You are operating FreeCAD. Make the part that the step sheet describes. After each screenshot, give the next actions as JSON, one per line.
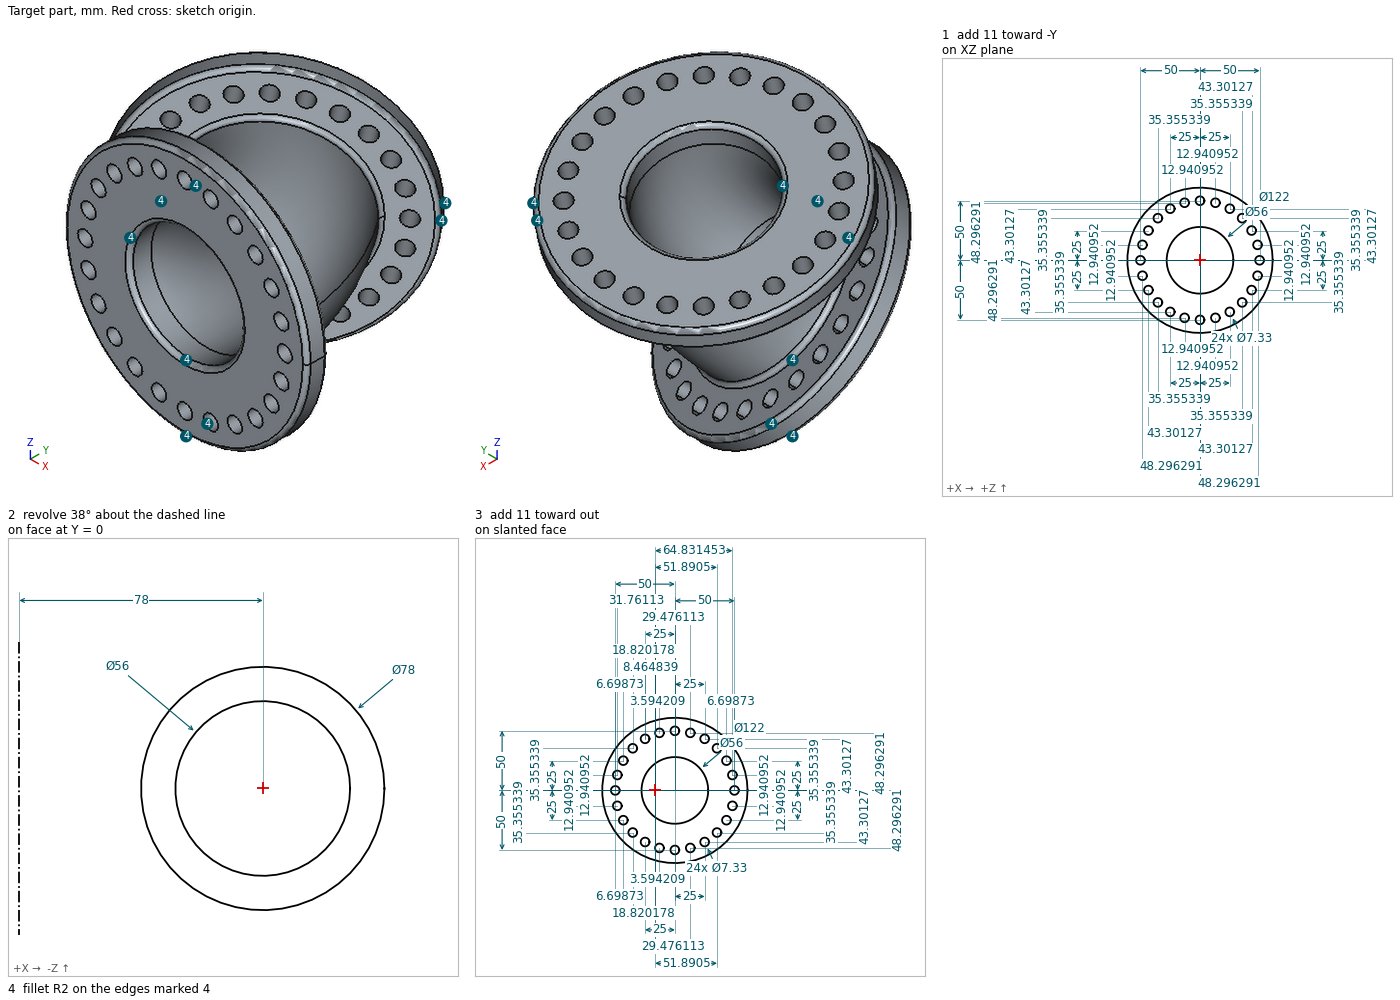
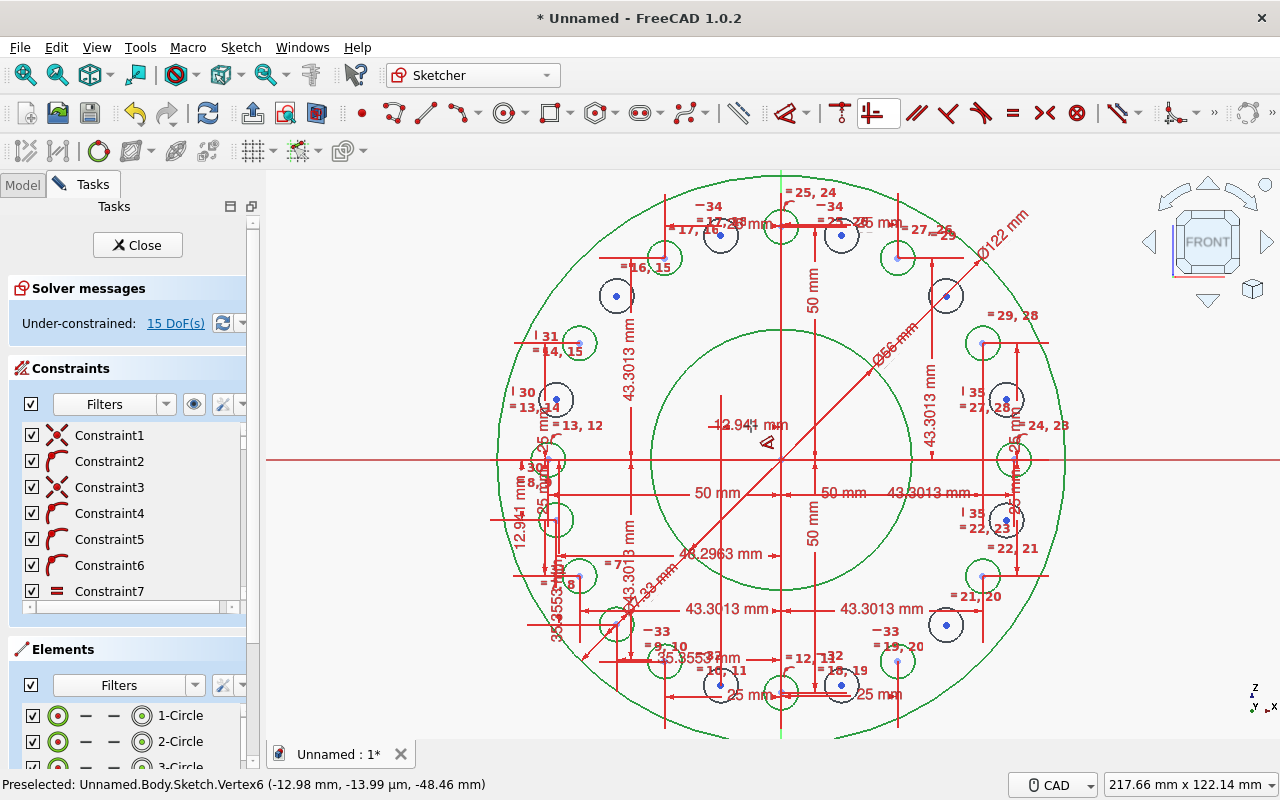
{"action": "left_click", "coordinate": [721, 686]}
{"action": "left_click", "coordinate": [687, 521]}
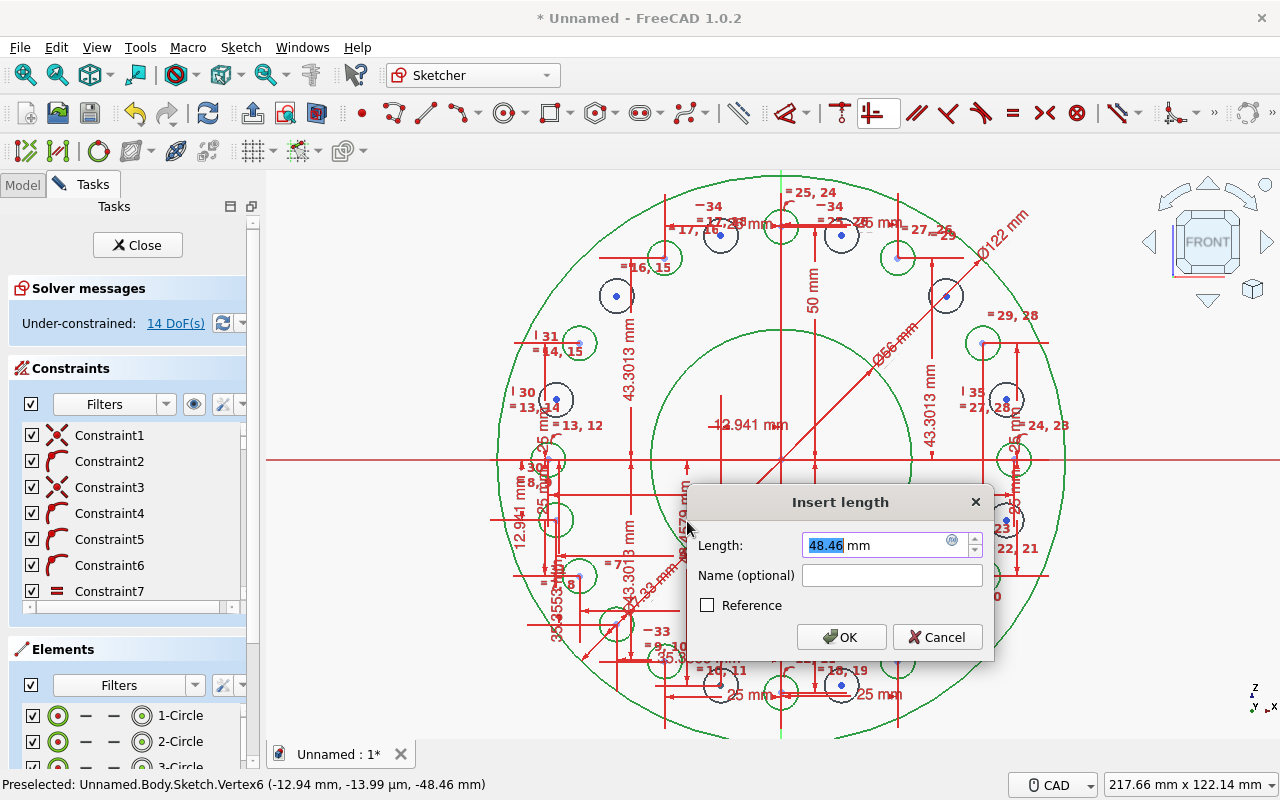
{"action": "type", "text": "48.296291"}
{"action": "key", "text": "Return"}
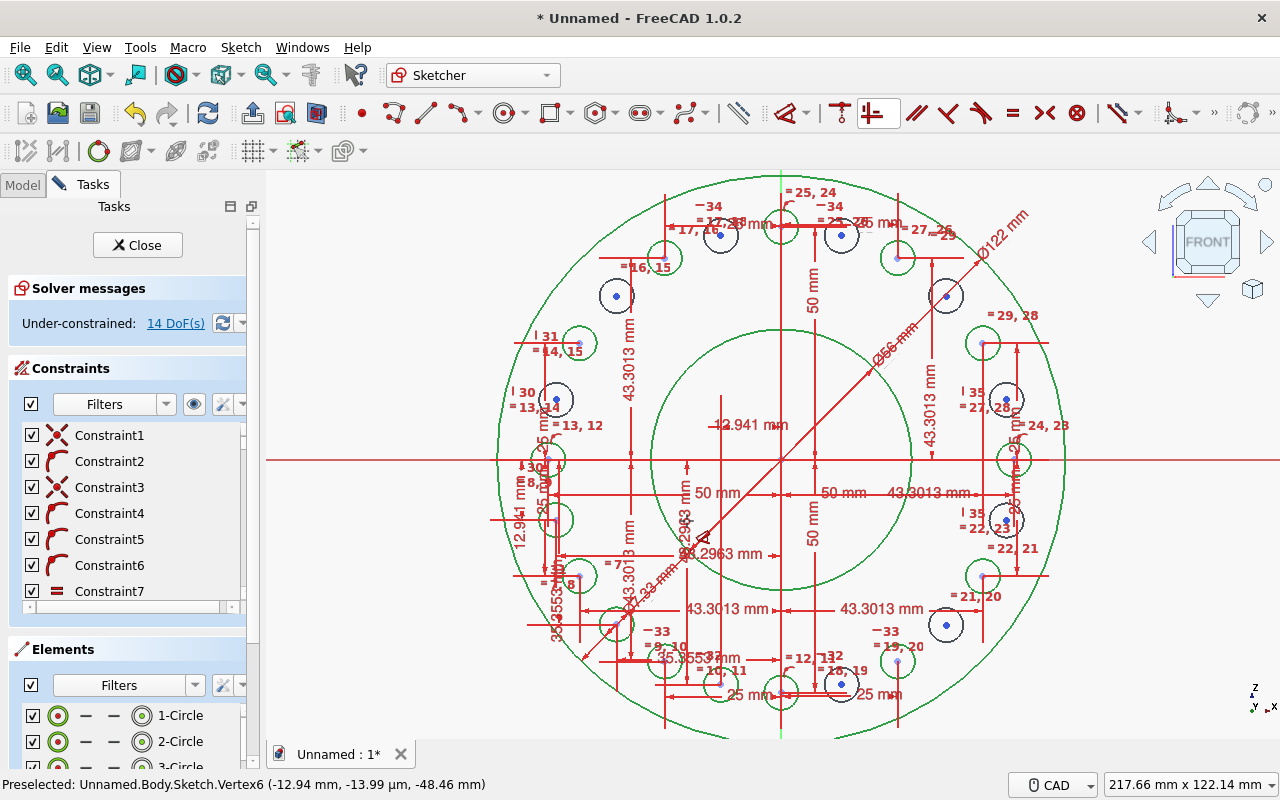
{"action": "left_click", "coordinate": [556, 400]}
{"action": "left_click", "coordinate": [839, 430]}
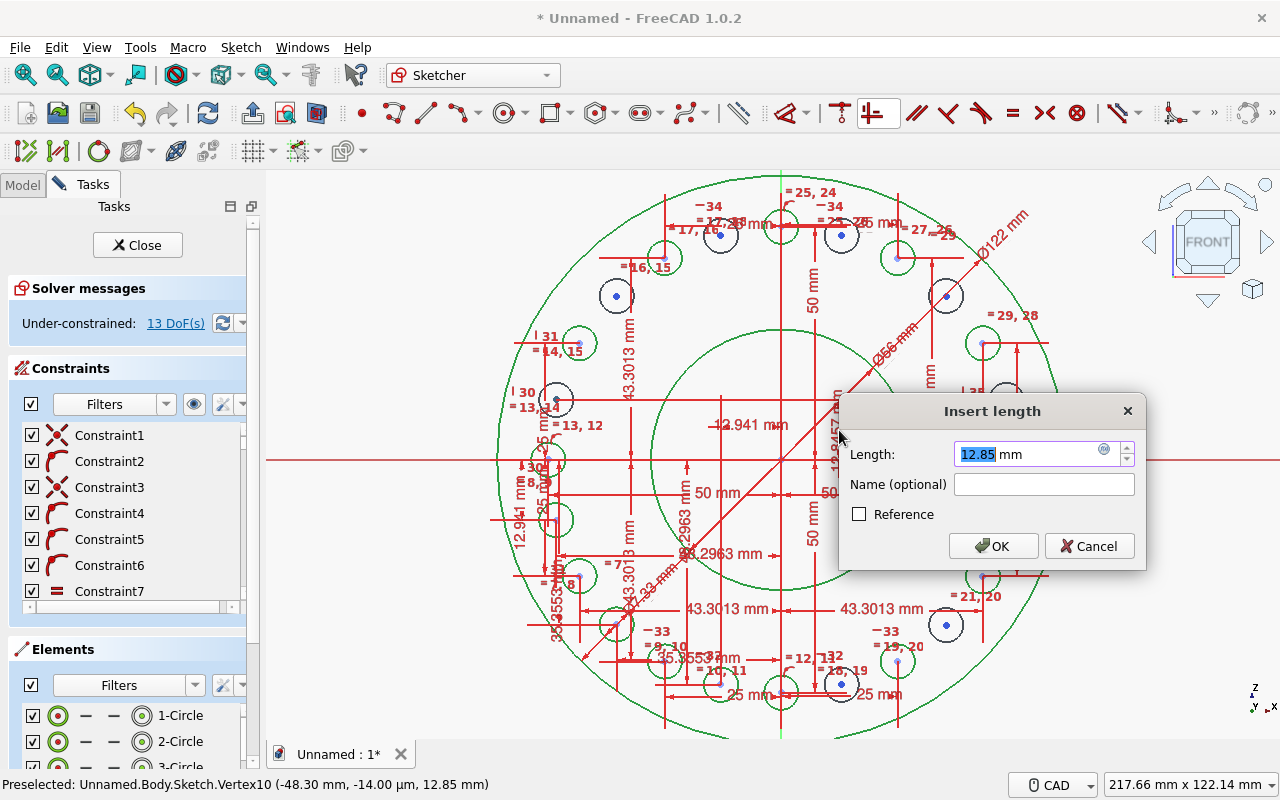
{"action": "type", "text": "12.940952"}
{"action": "key", "text": "Return"}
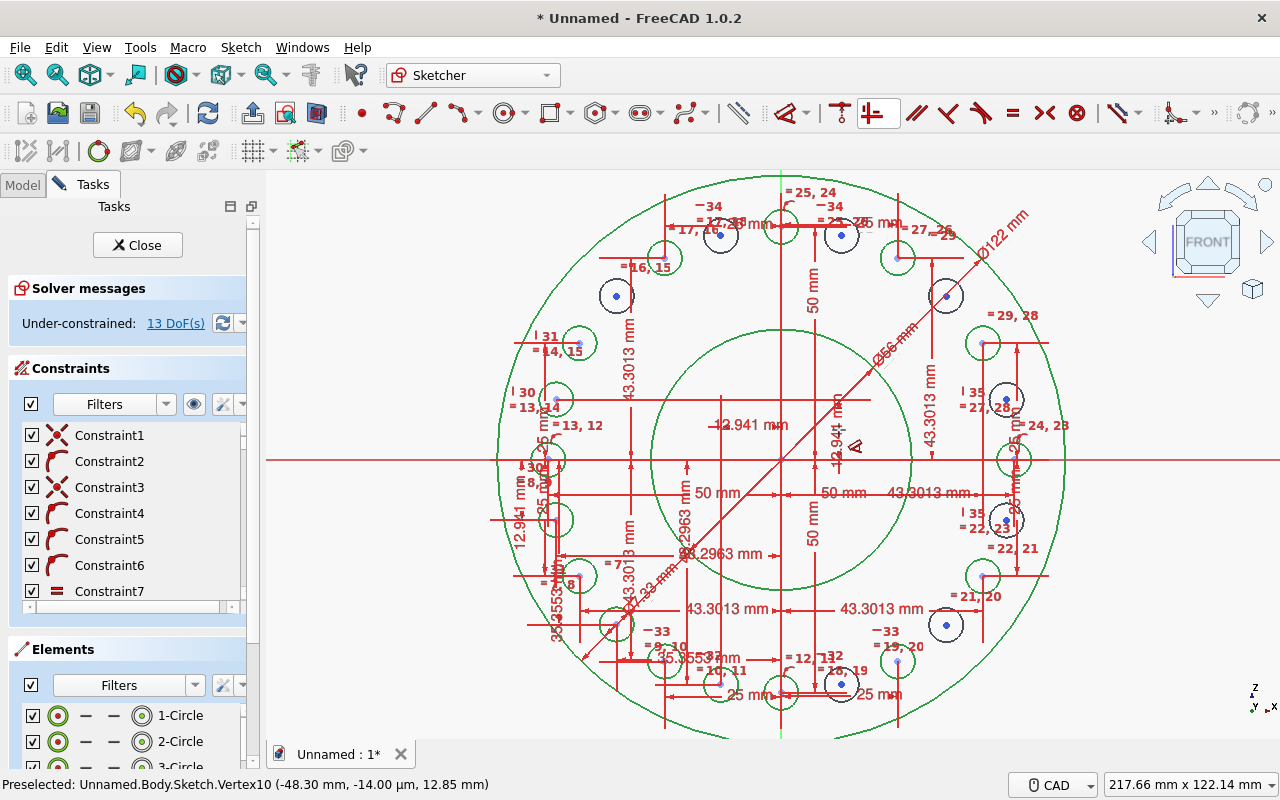
{"action": "left_click", "coordinate": [617, 296]}
{"action": "left_click", "coordinate": [699, 262]}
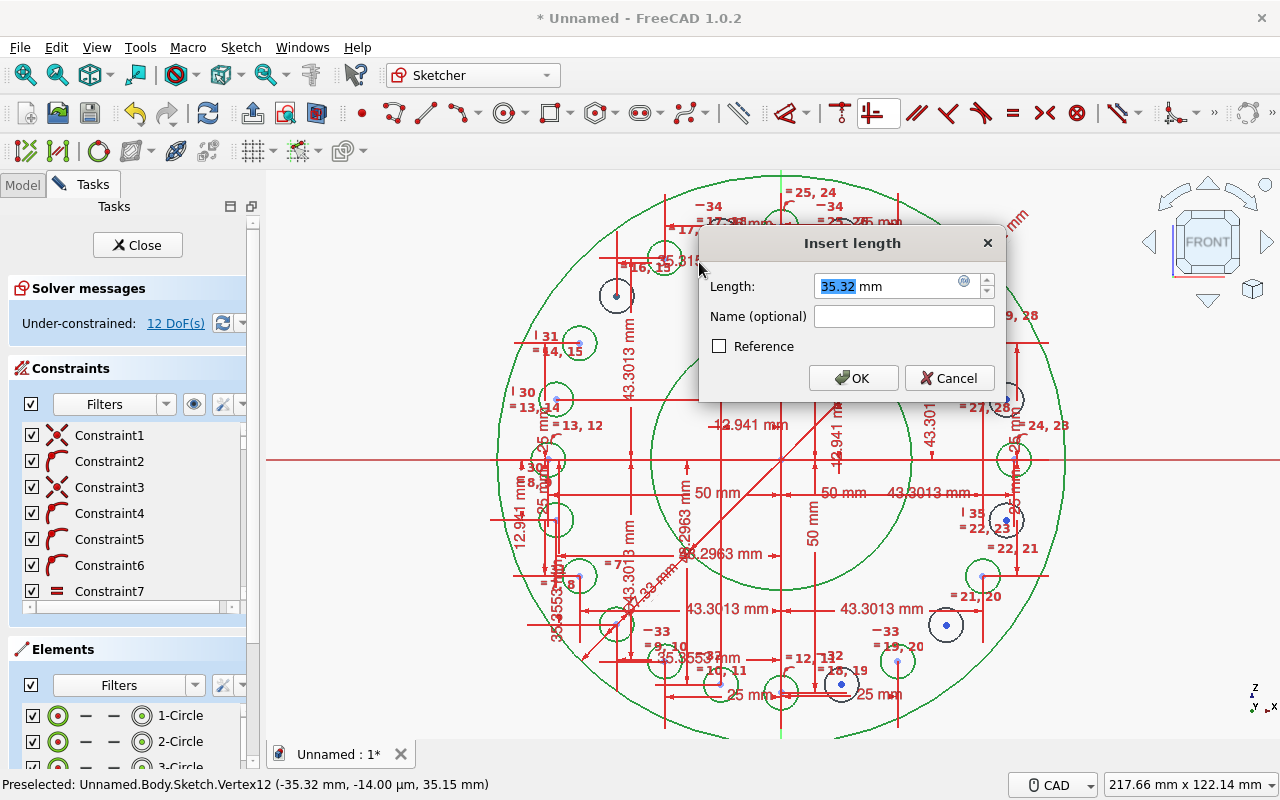
{"action": "type", "text": "35.355339"}
{"action": "key", "text": "Return"}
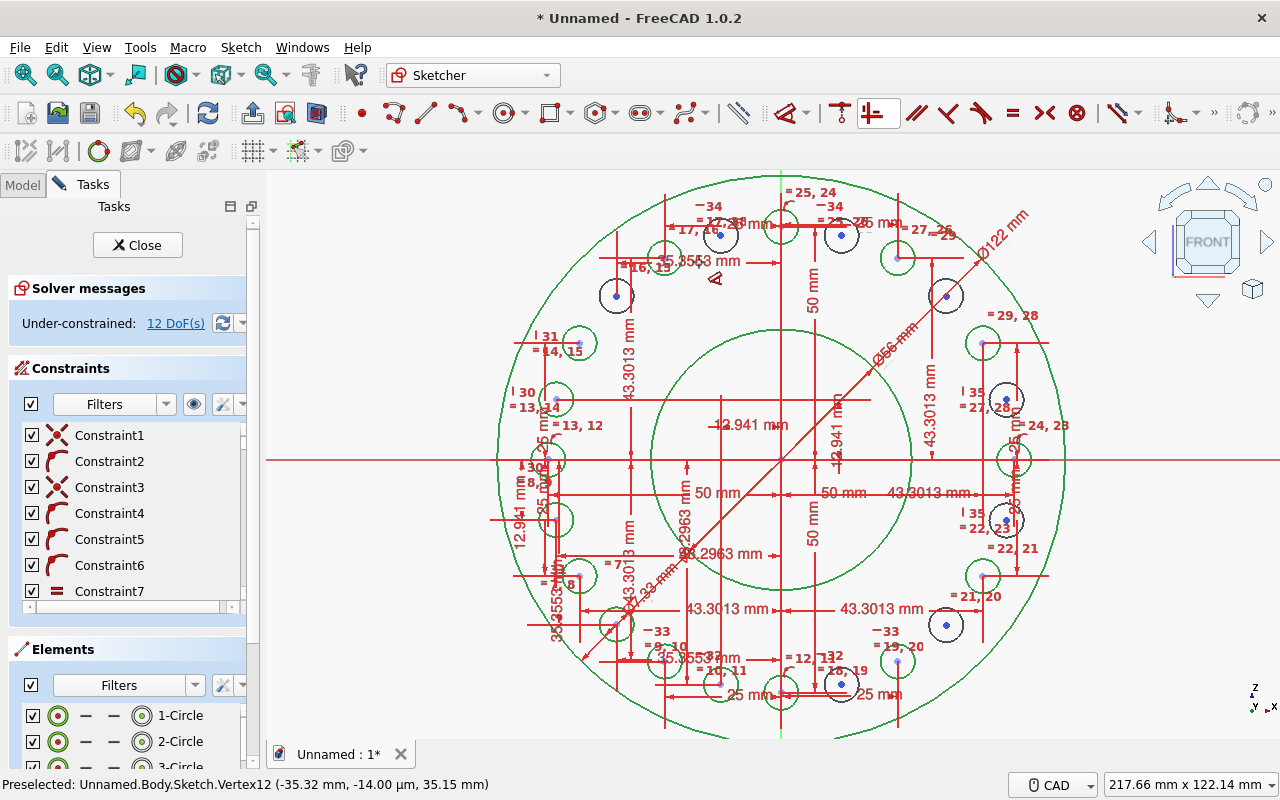
{"action": "left_click", "coordinate": [617, 296]}
{"action": "left_click", "coordinate": [815, 378]}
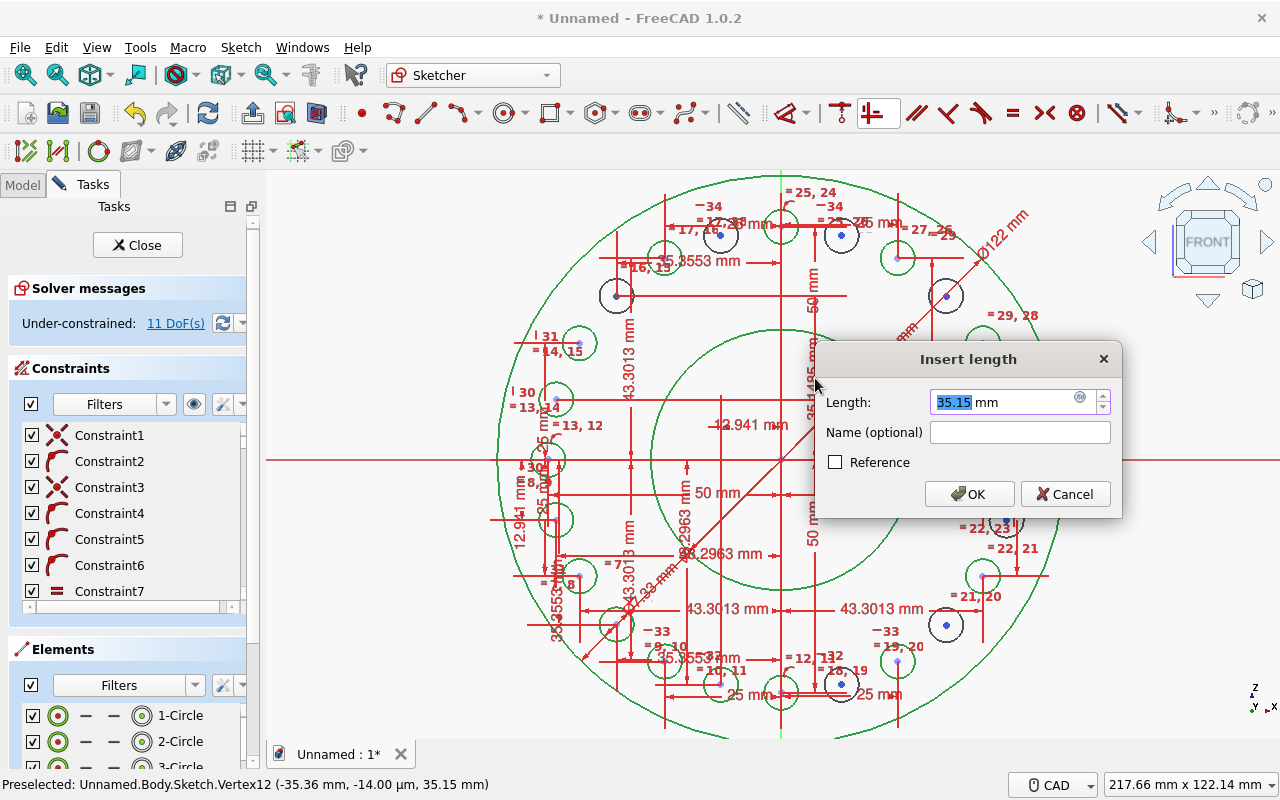
{"action": "type", "text": "35.355339"}
{"action": "key", "text": "Return"}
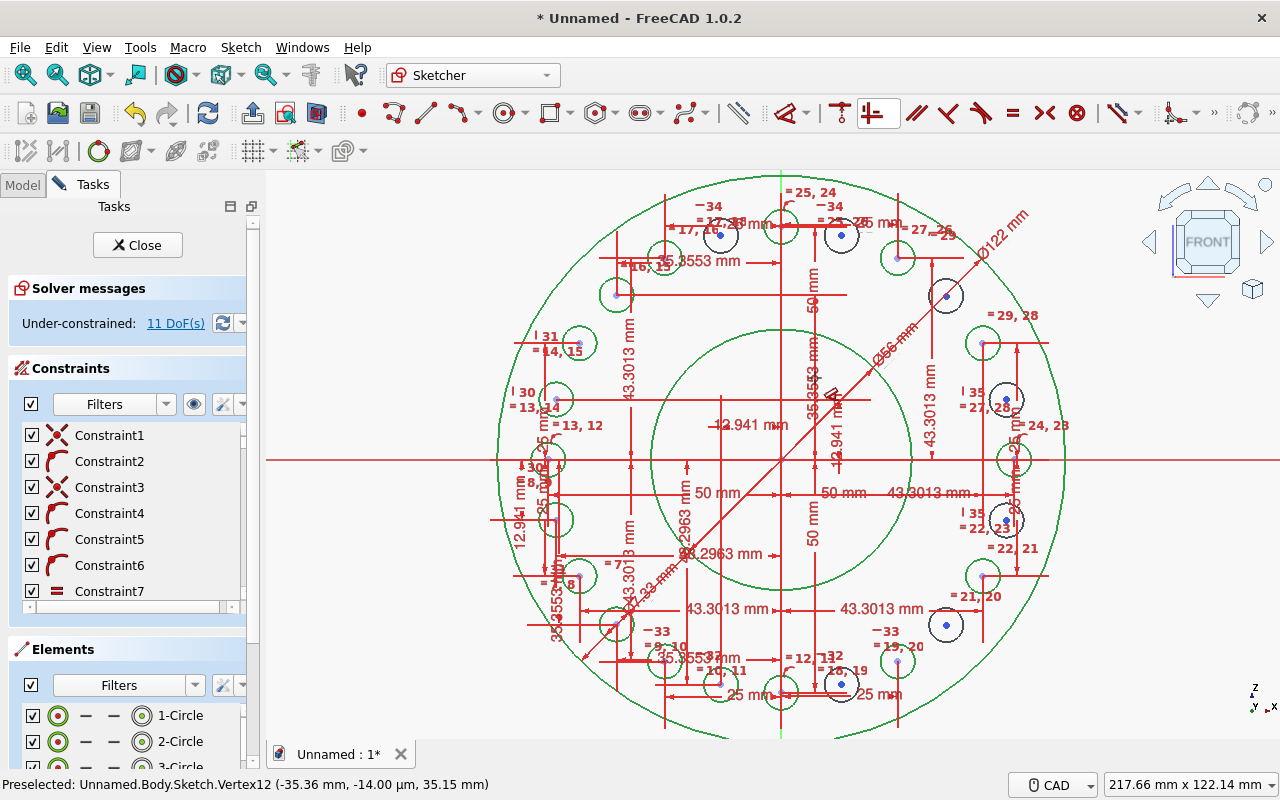
{"action": "left_click", "coordinate": [721, 236]}
{"action": "left_click", "coordinate": [751, 202]}